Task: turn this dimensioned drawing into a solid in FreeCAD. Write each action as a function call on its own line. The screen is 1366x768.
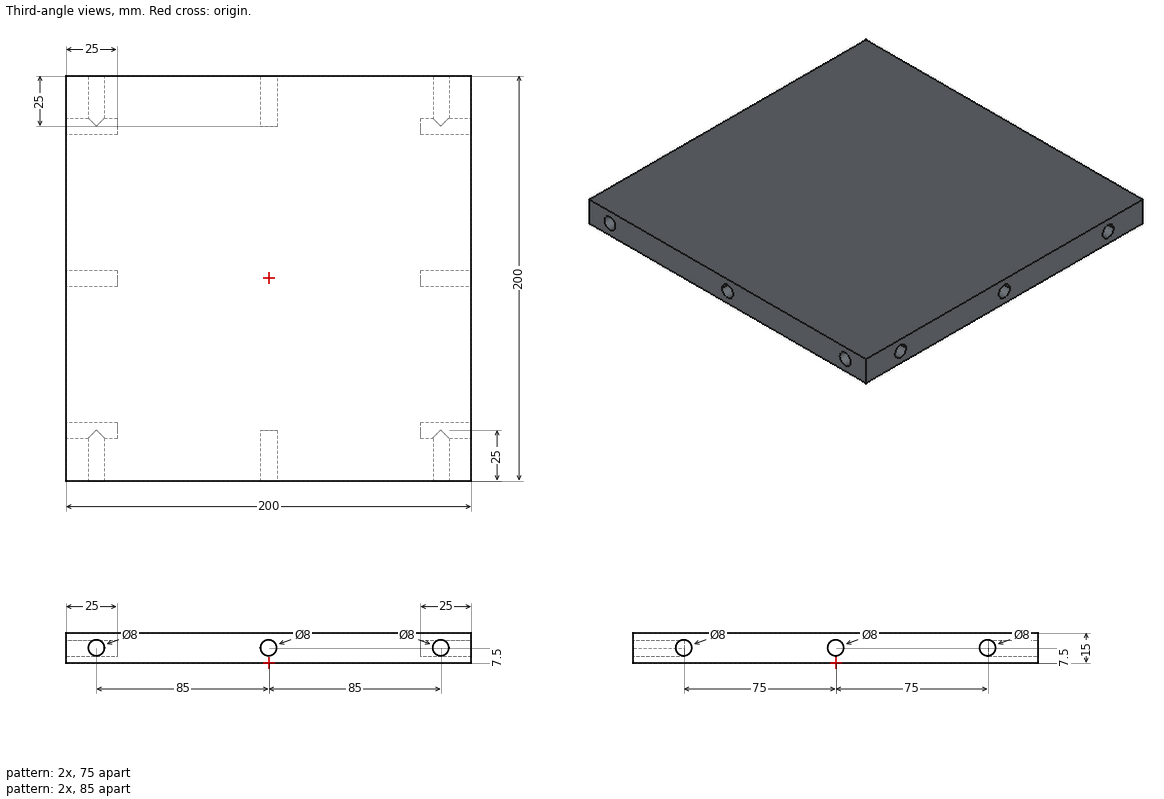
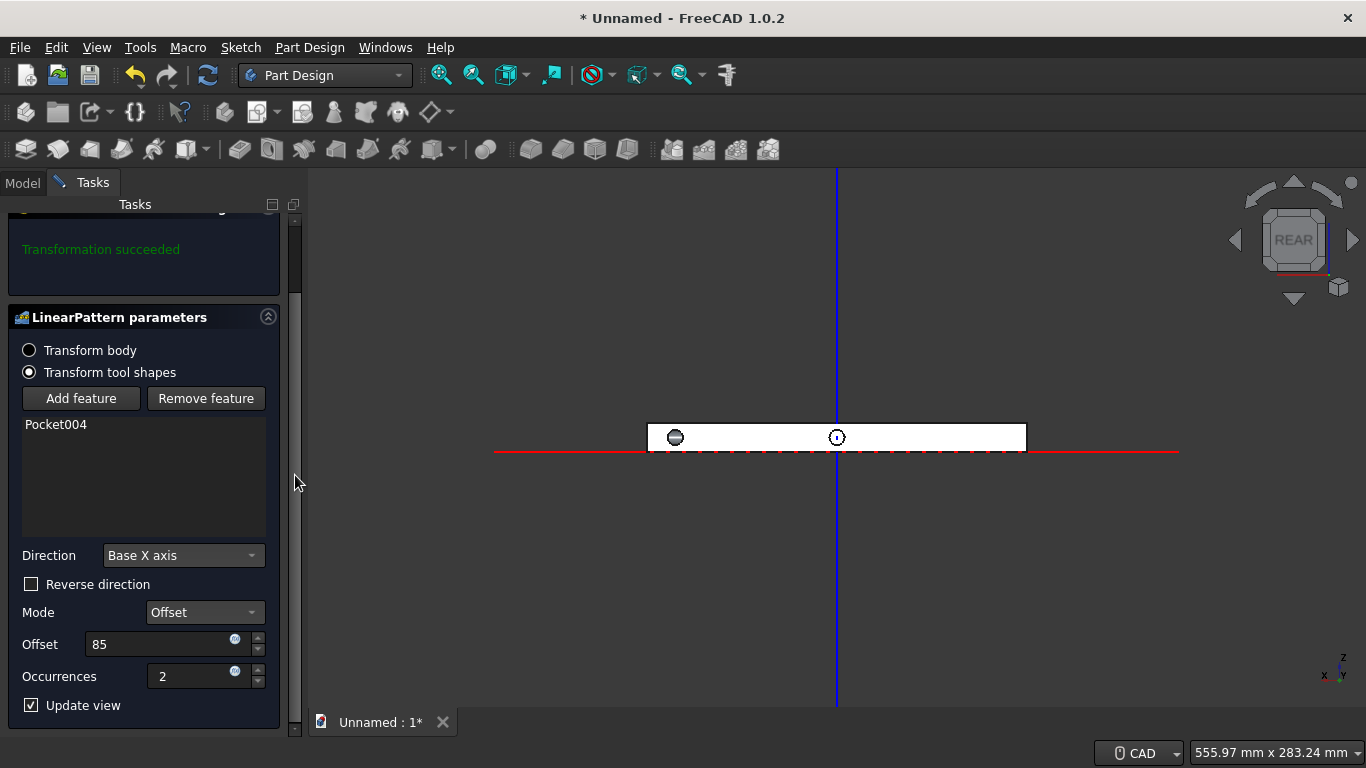
triple_click(198, 676)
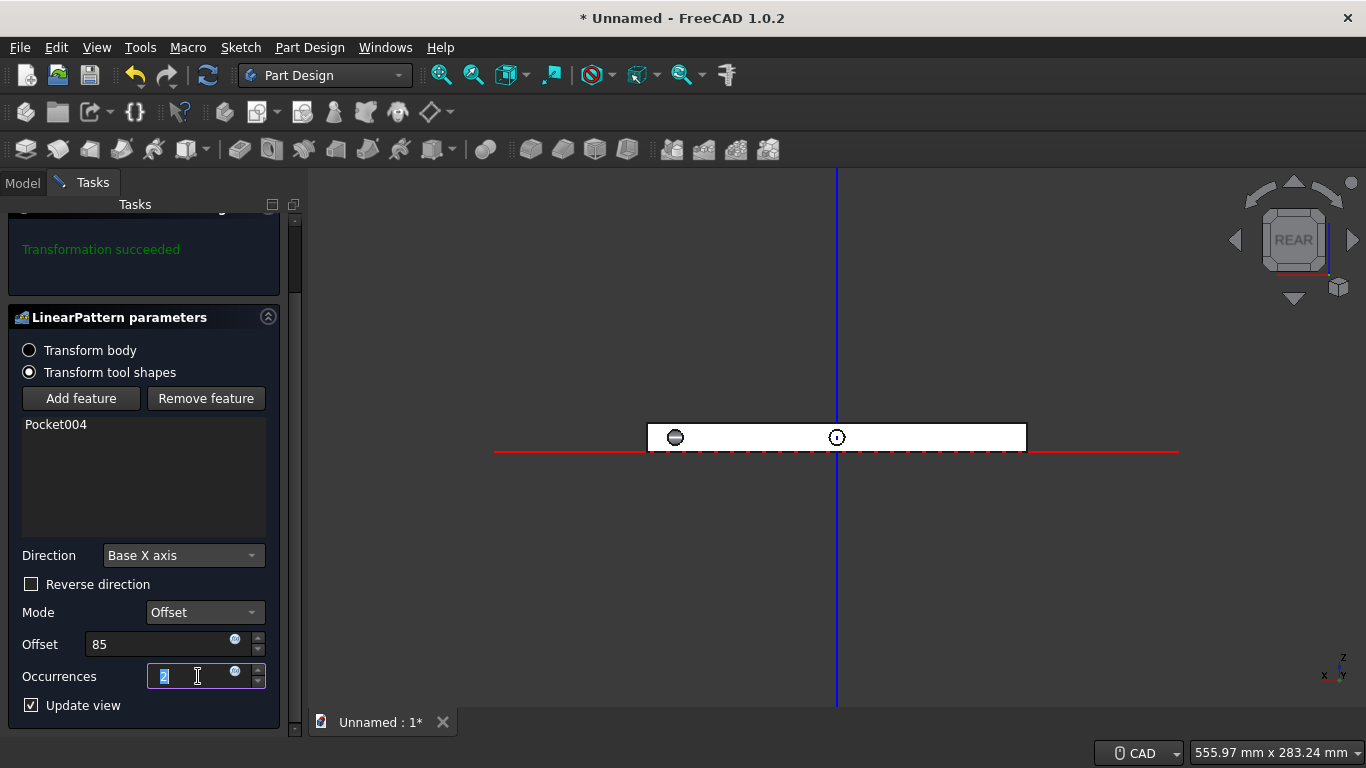
text(2)
key(Tab)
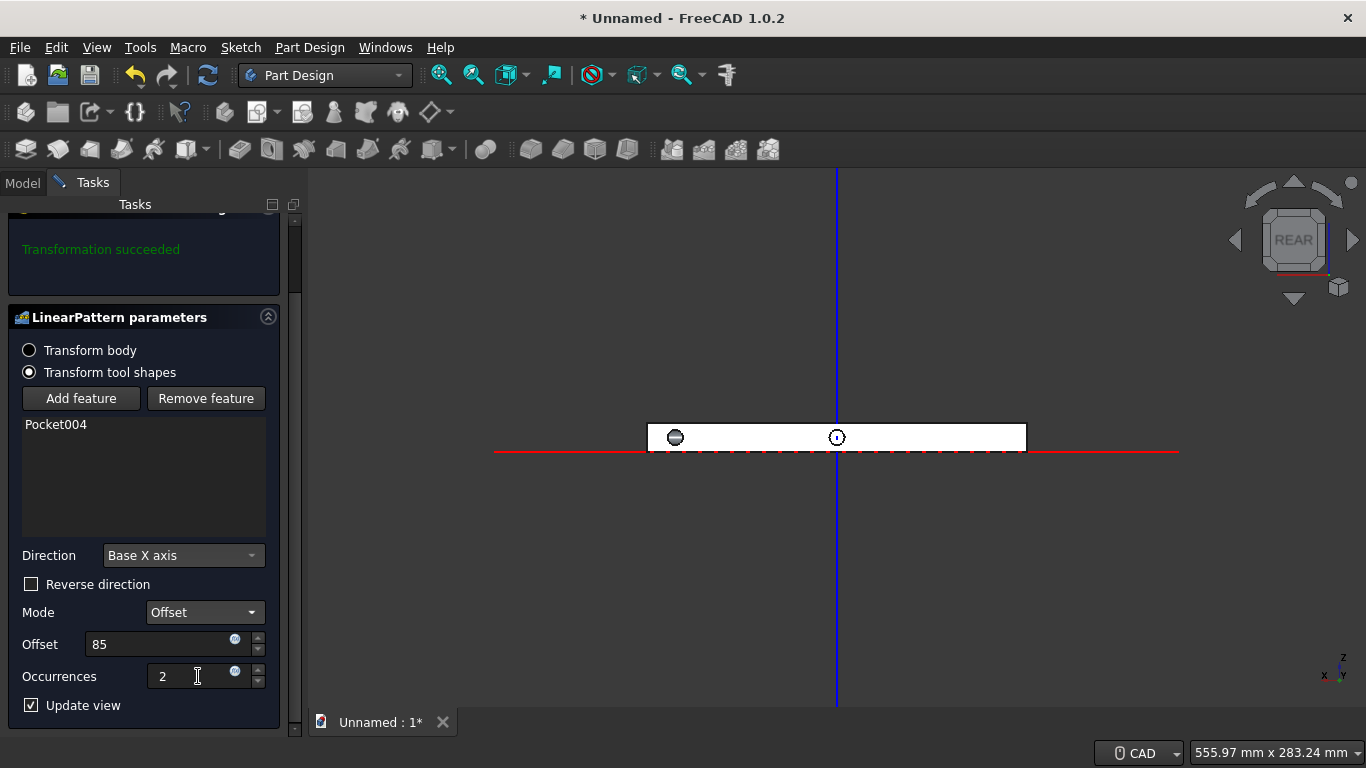
scroll(295, 475, up, 3)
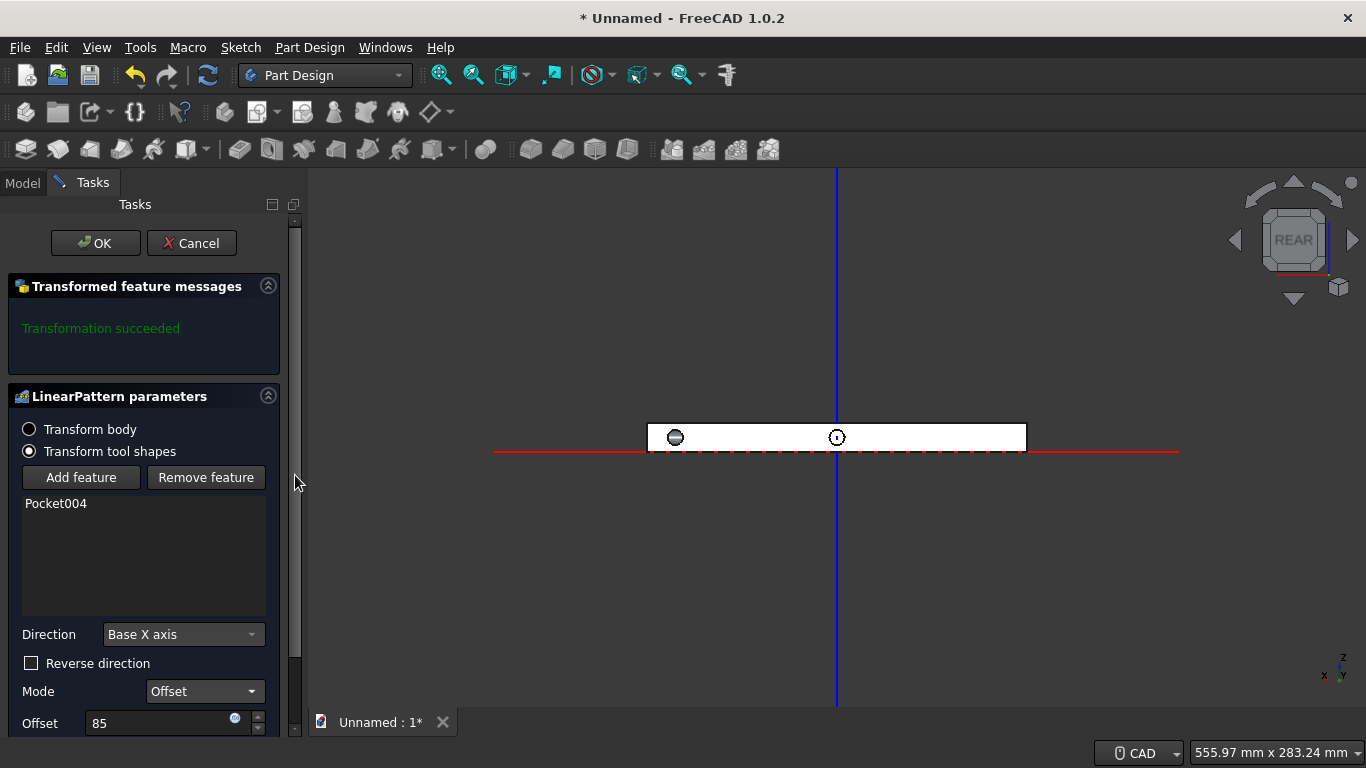
click(96, 243)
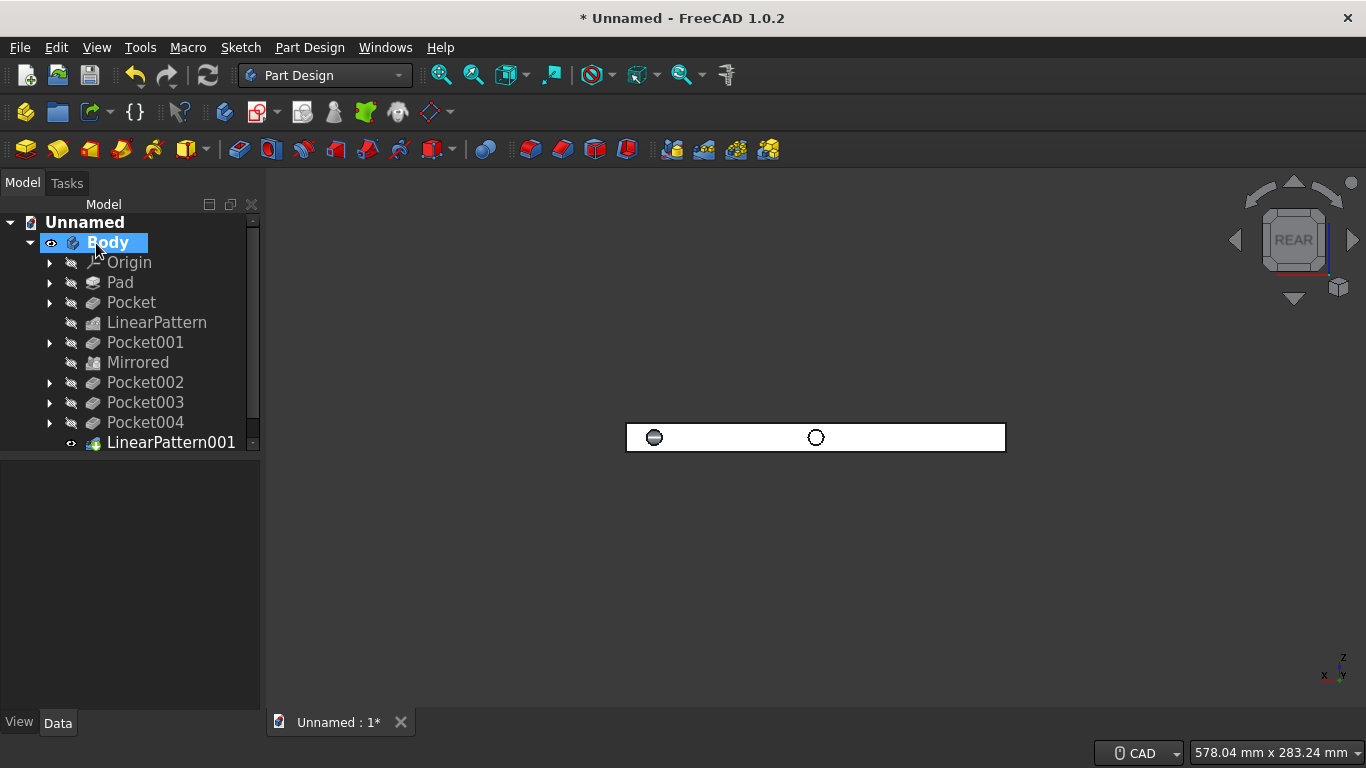
key(v)
key(f)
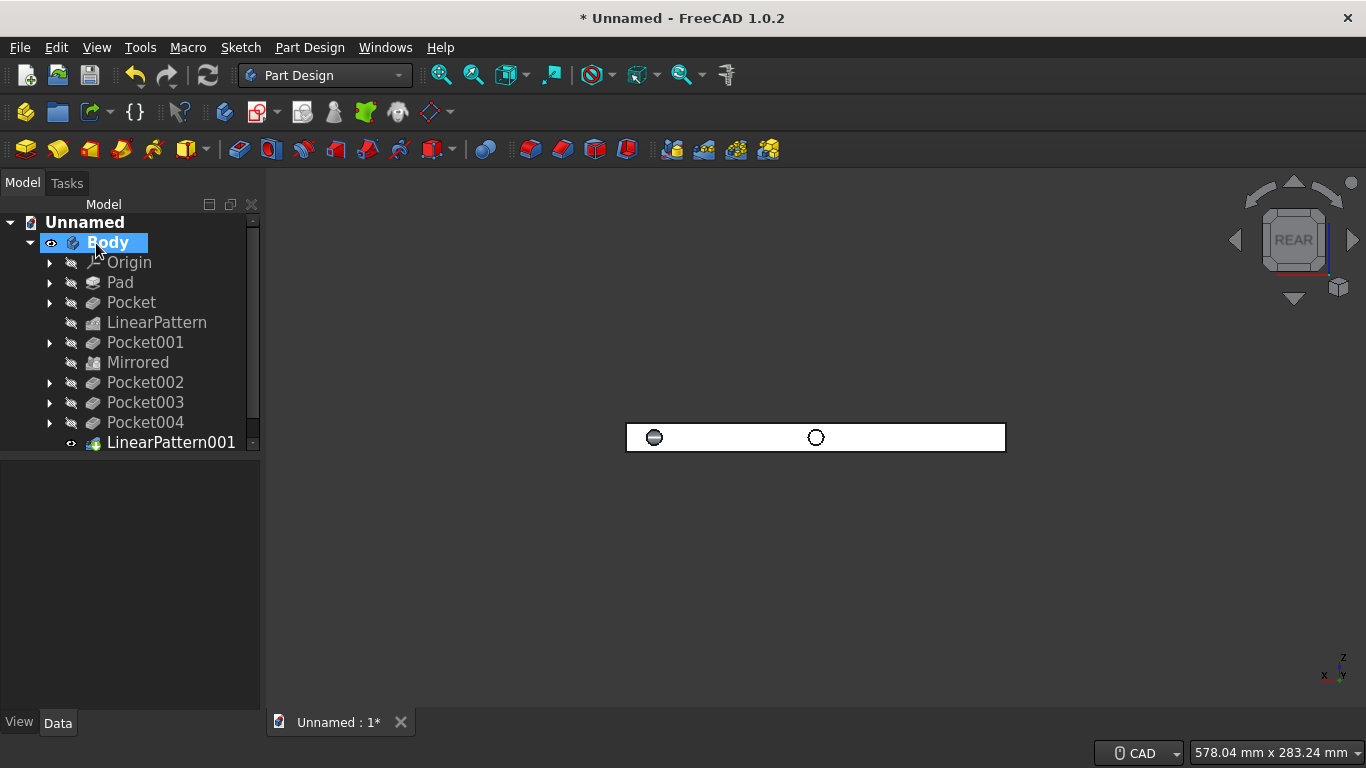
click(707, 436)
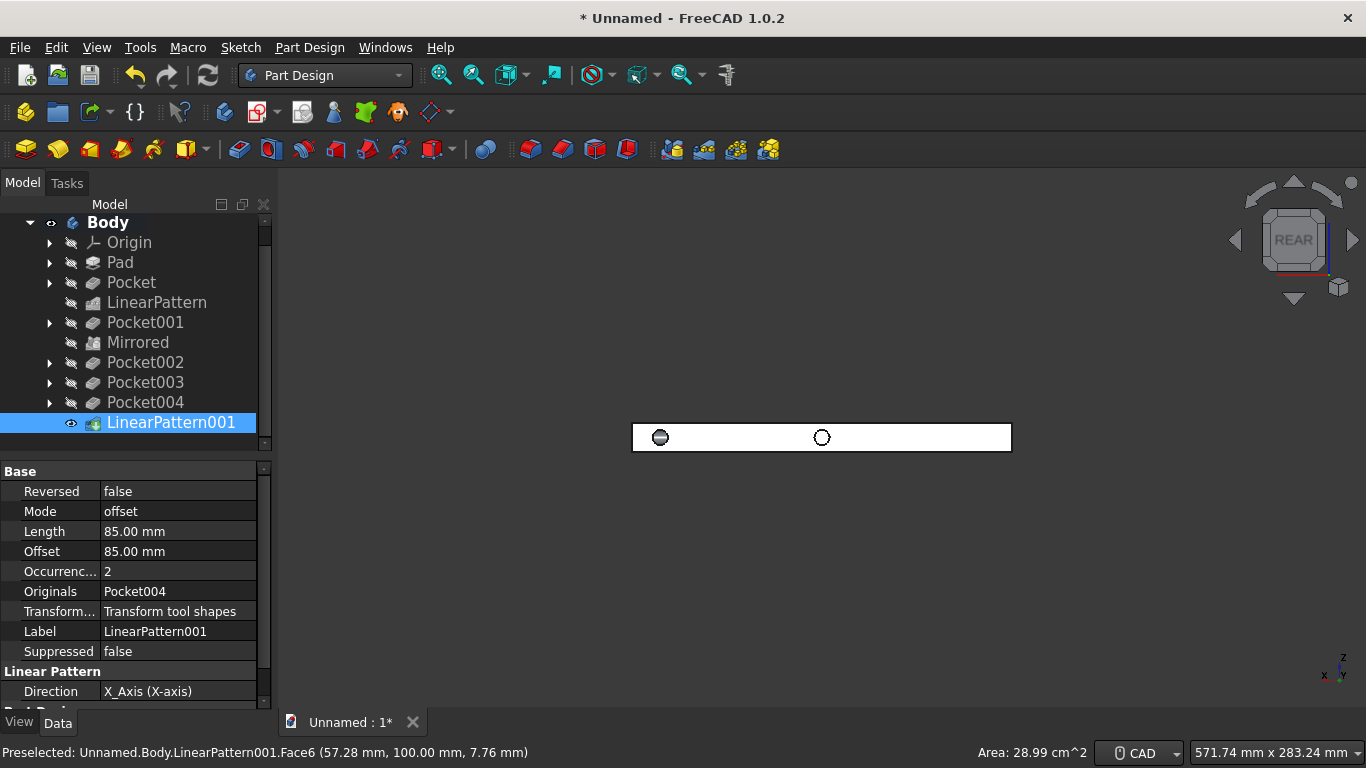
click(258, 112)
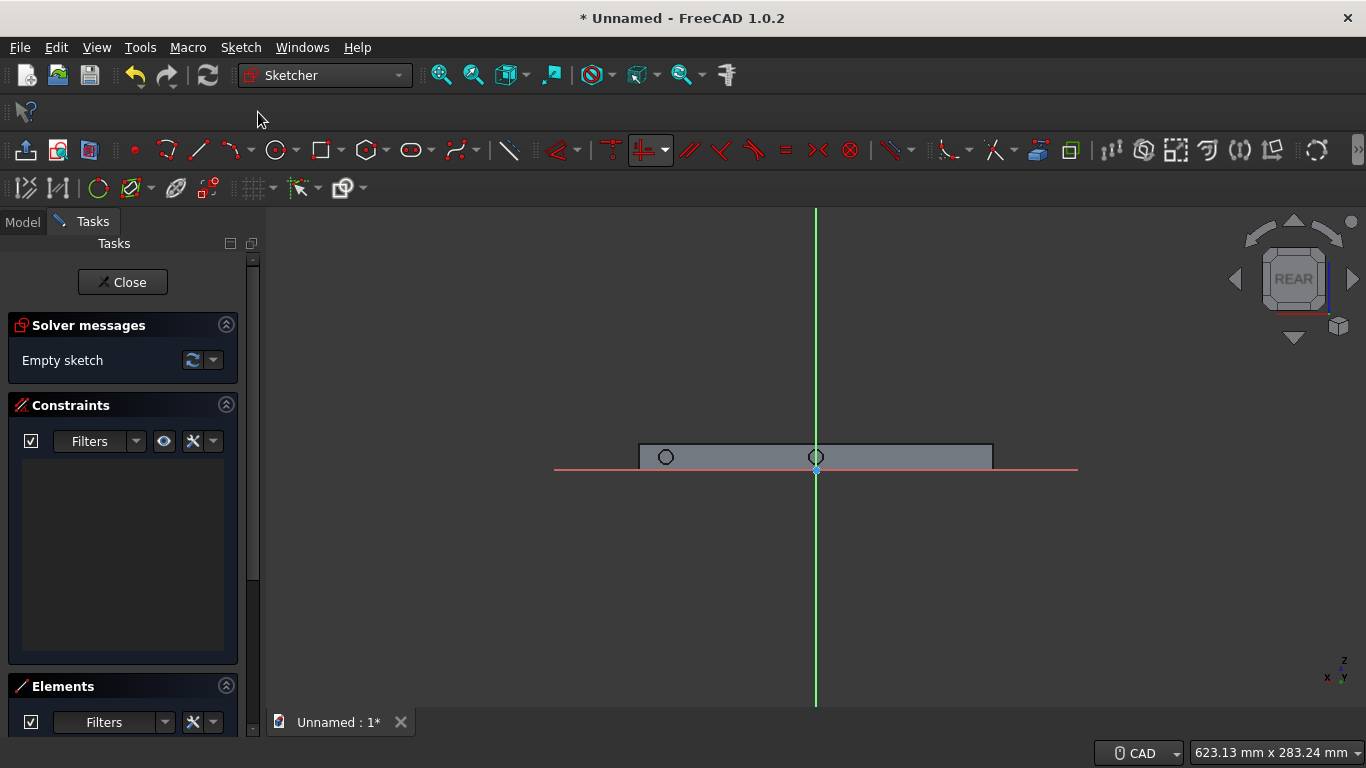
scroll(978, 457, up, 15)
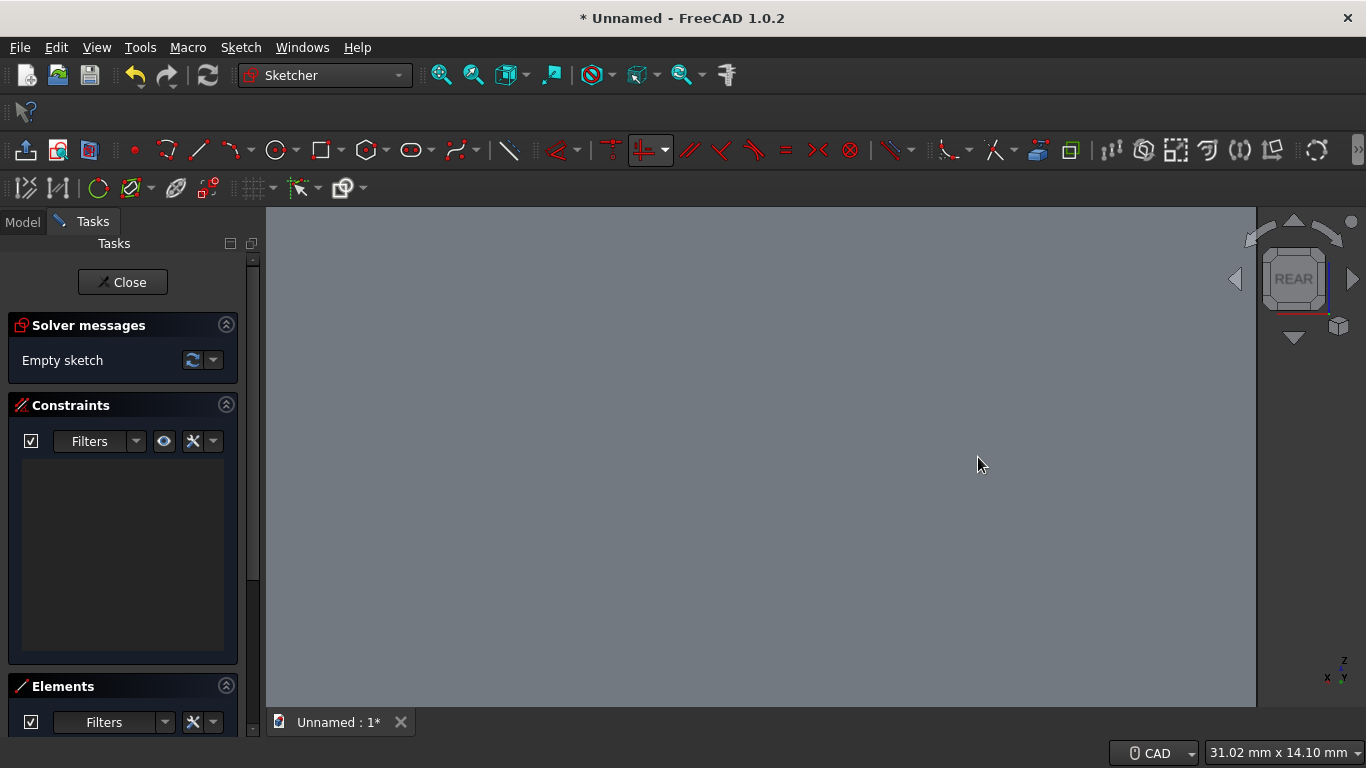
key(g)
key(c)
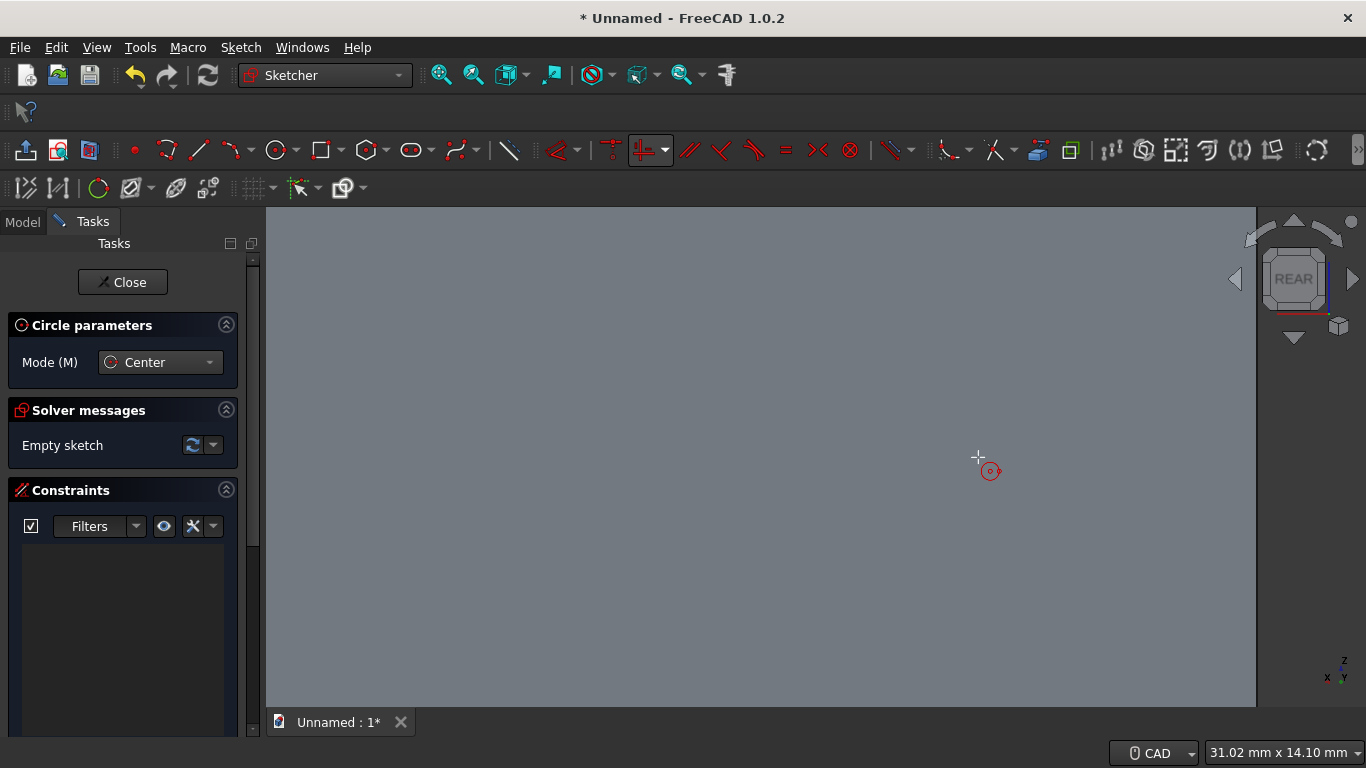
click(726, 447)
move(826, 347)